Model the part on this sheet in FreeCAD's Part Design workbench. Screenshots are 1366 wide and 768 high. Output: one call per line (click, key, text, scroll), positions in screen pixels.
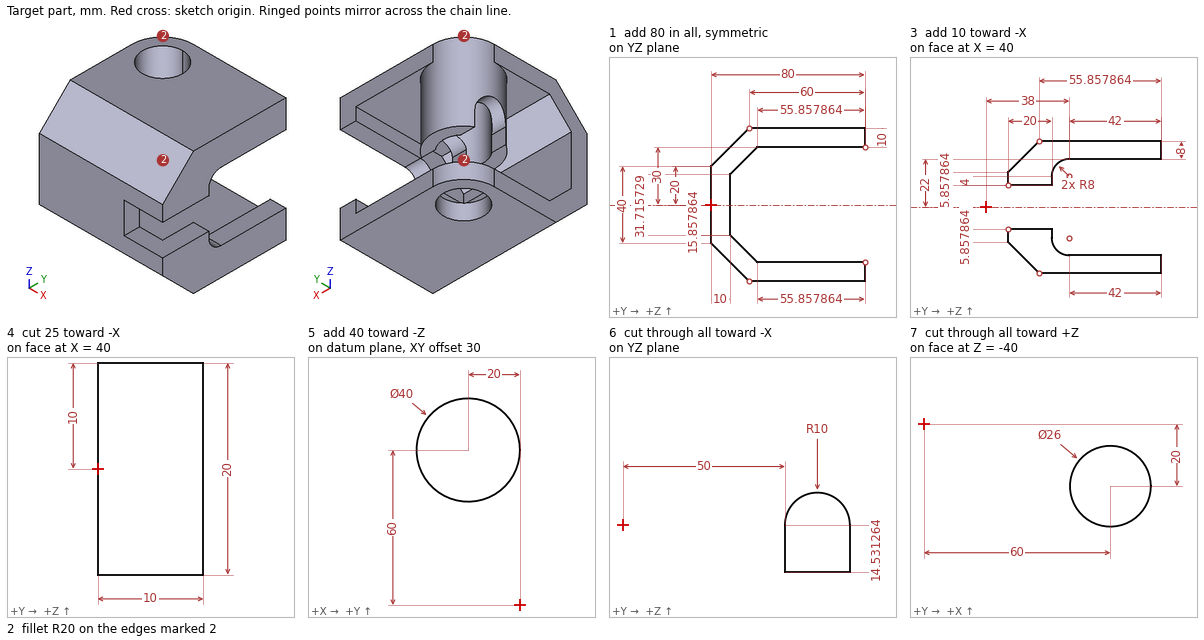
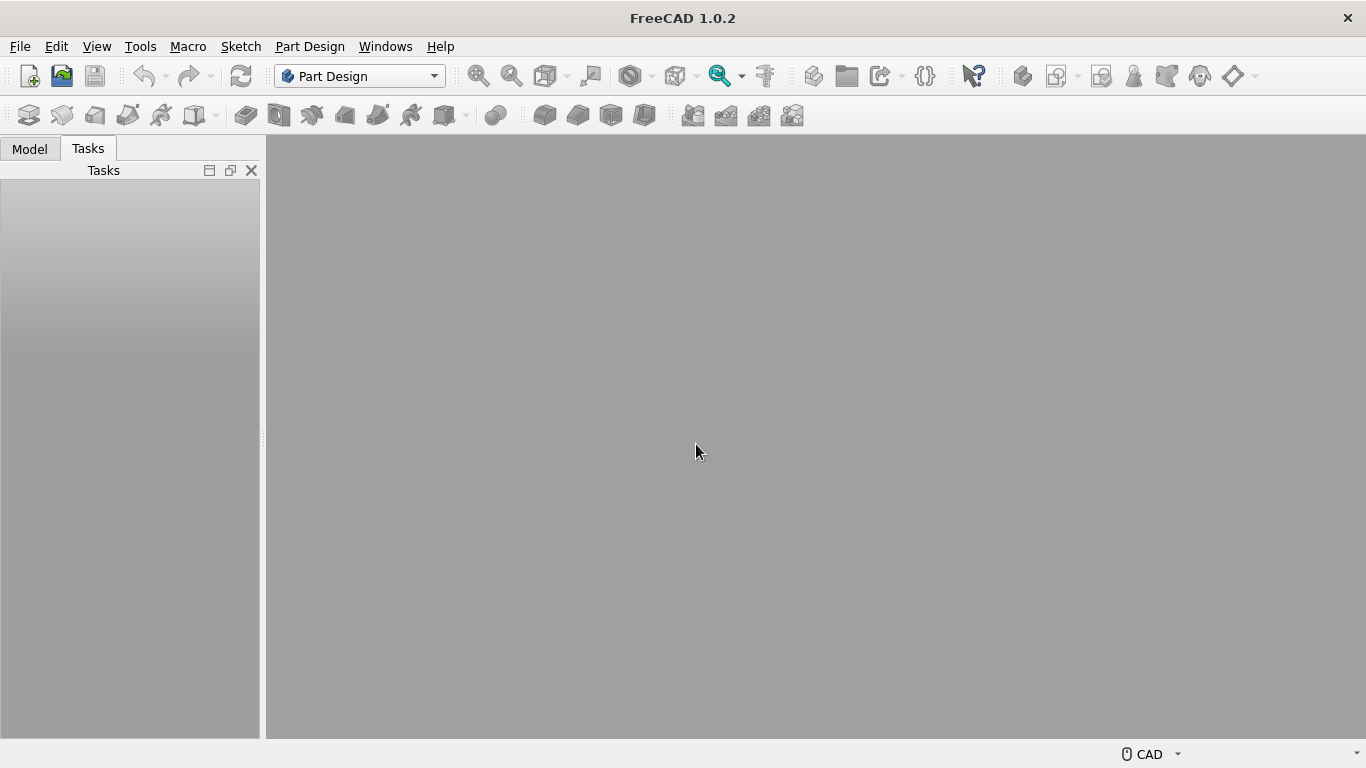
key(ctrl+n)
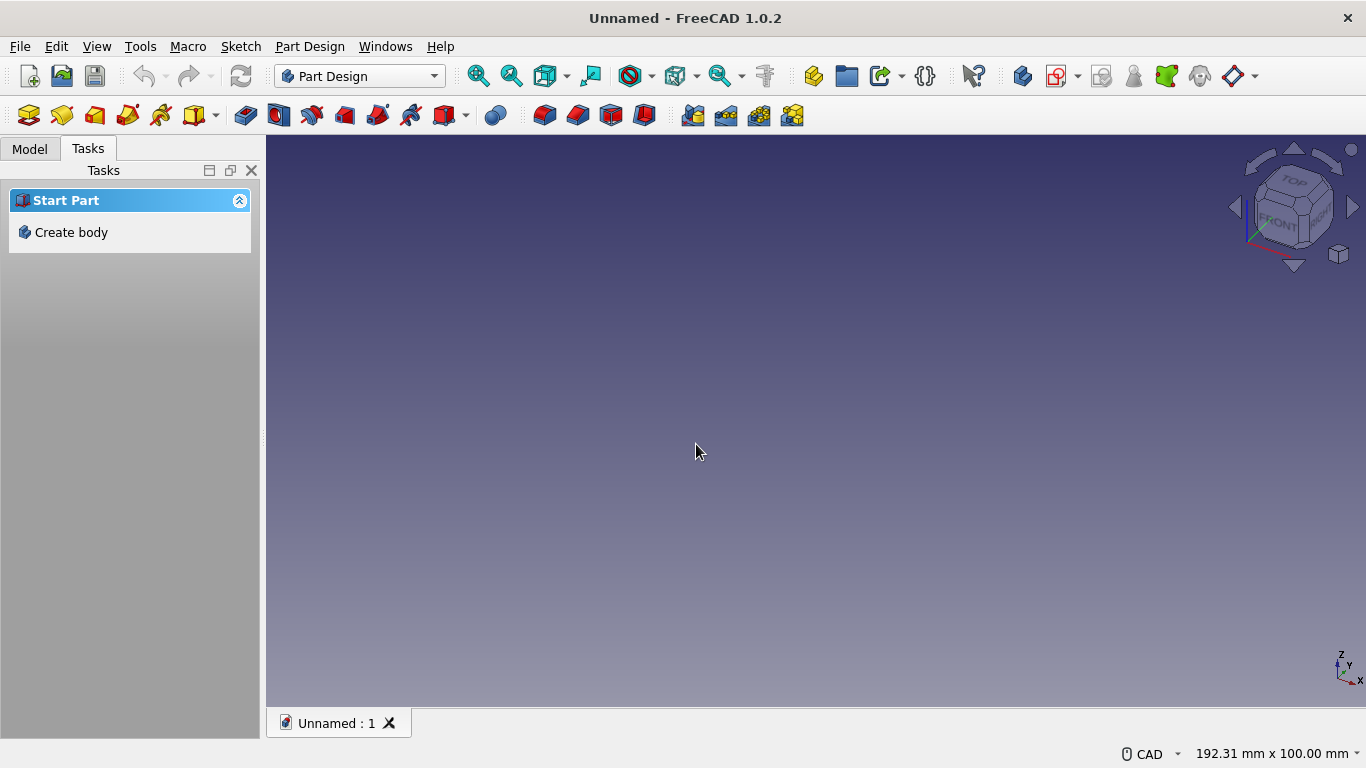
click(1056, 76)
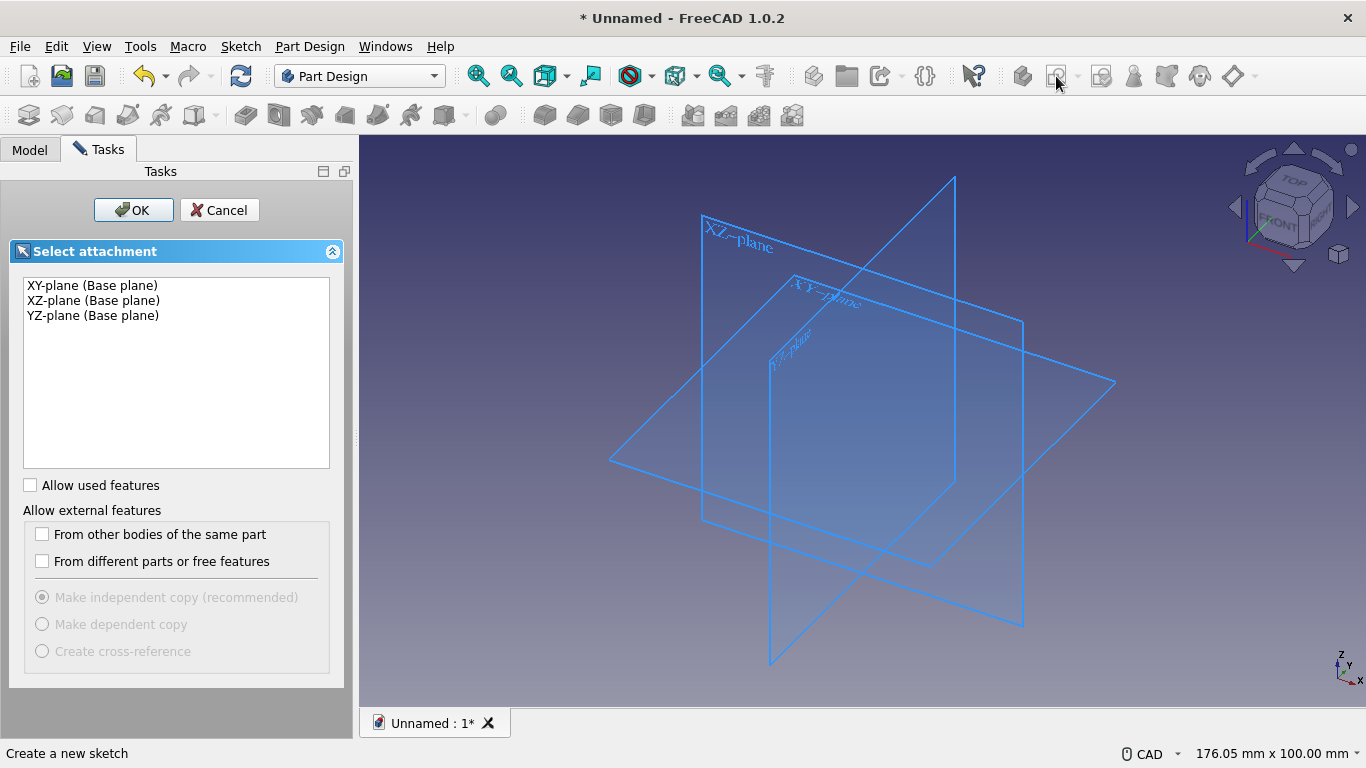
click(84, 316)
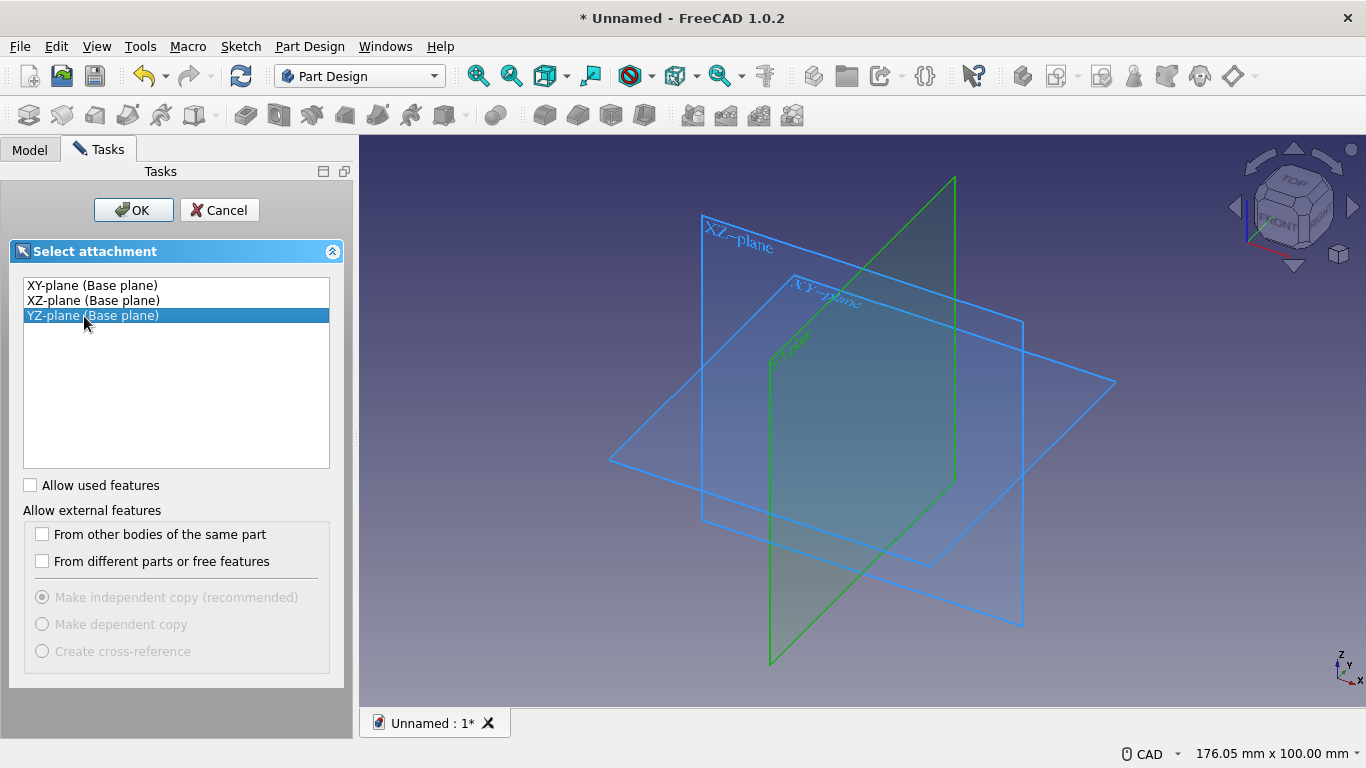
click(134, 210)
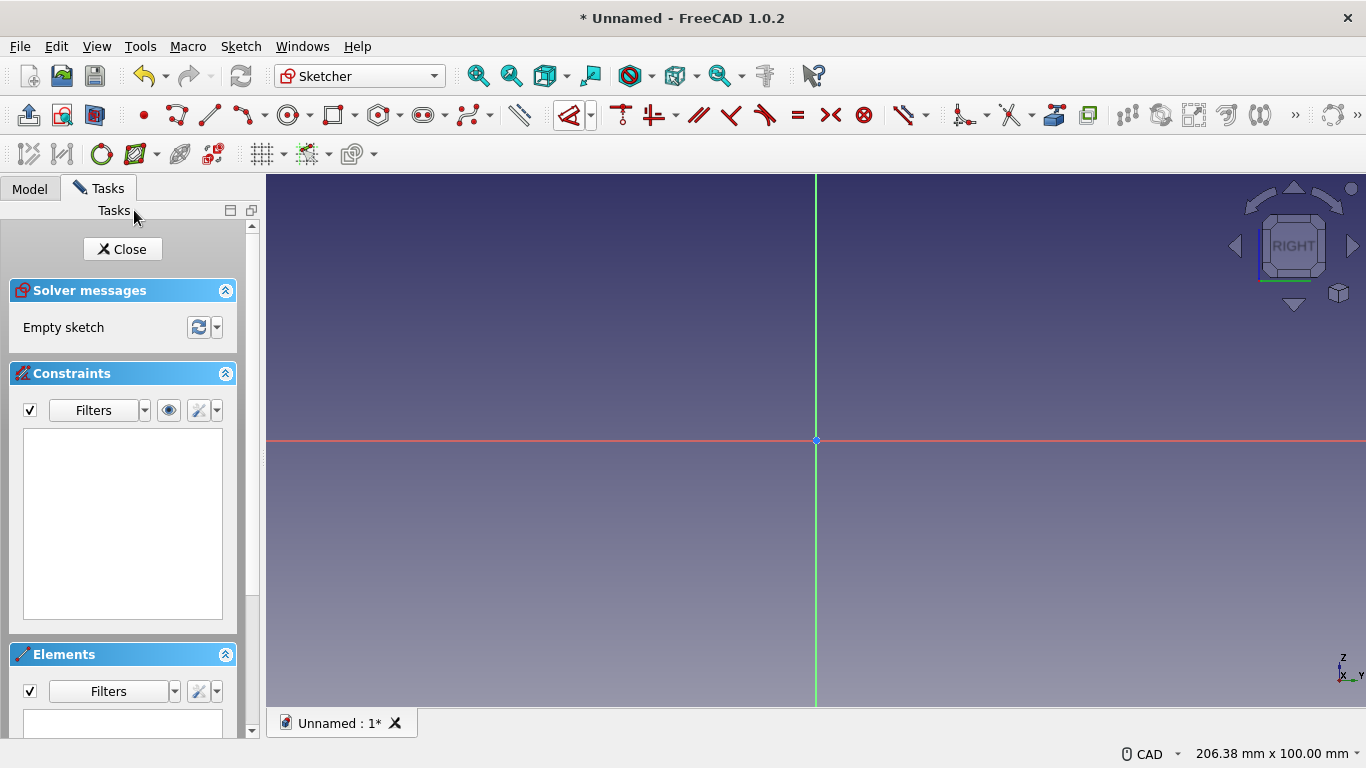
scroll(294, 440, down, 1)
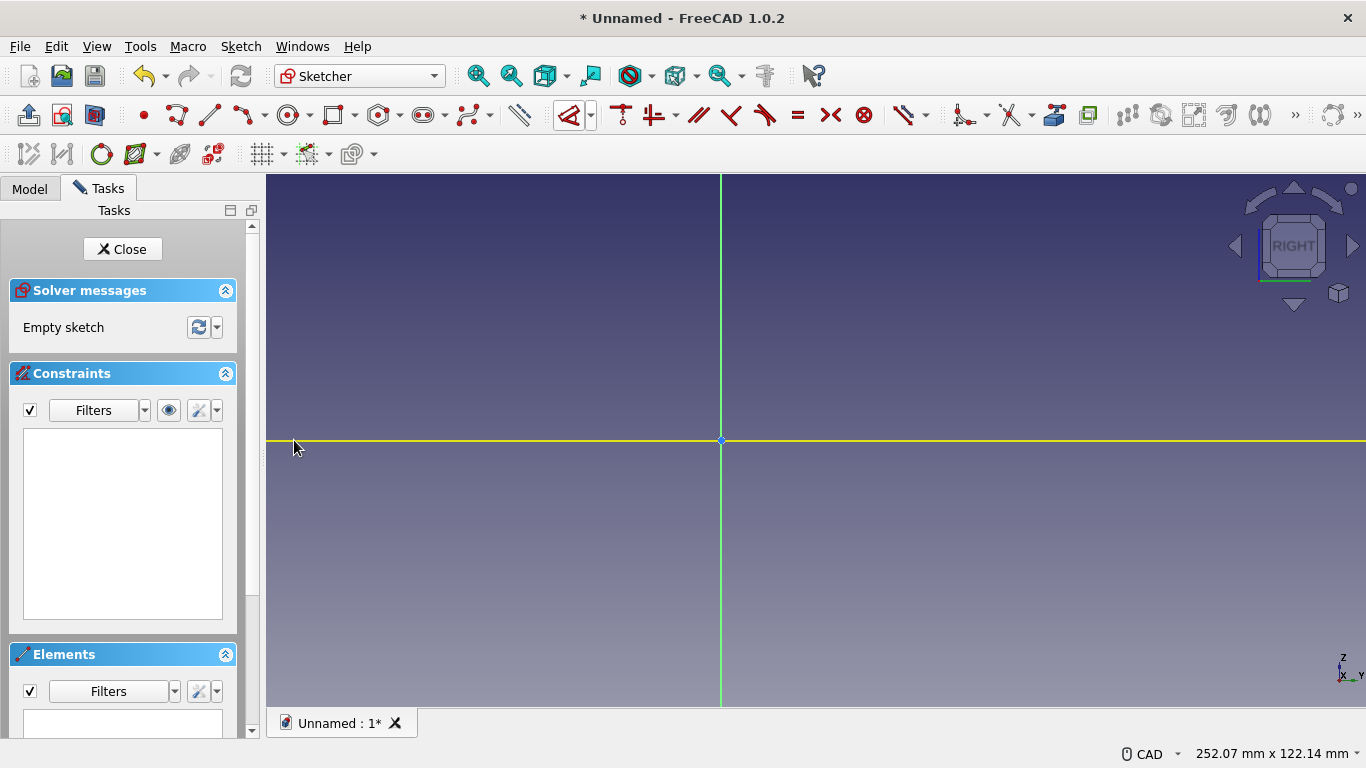
click(177, 116)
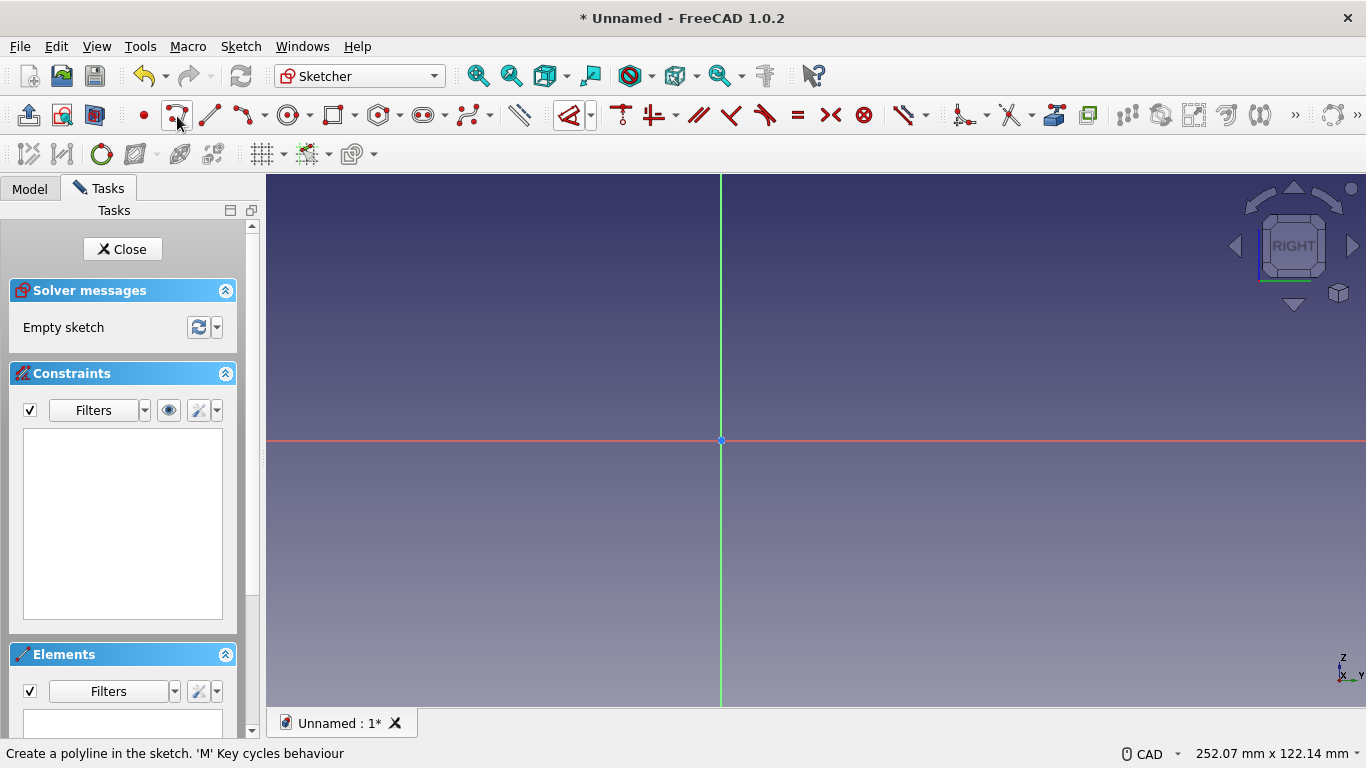
click(765, 510)
click(765, 371)
click(827, 310)
click(1070, 310)
click(1070, 266)
click(809, 266)
click(721, 353)
click(730, 528)
click(809, 615)
click(1070, 615)
click(1070, 571)
click(827, 571)
click(765, 511)
key(Escape)
key(Escape)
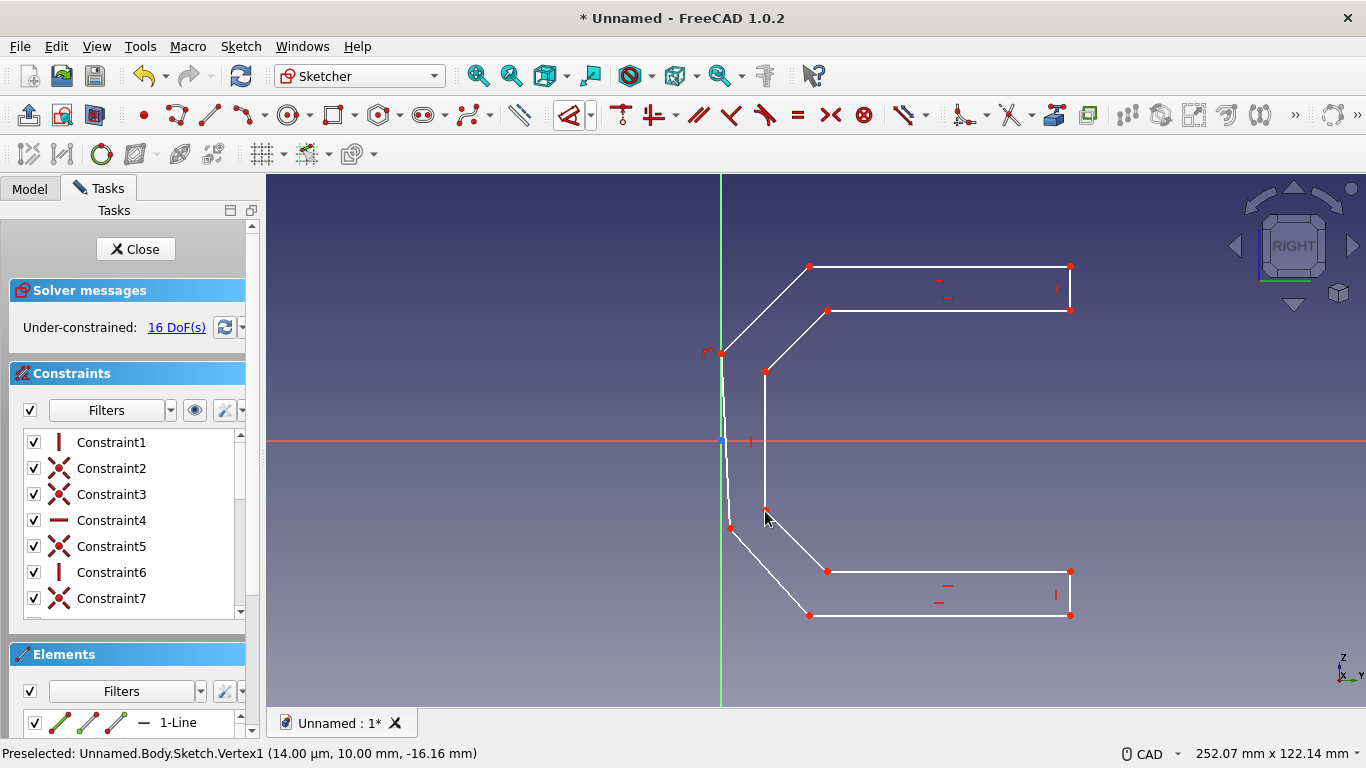
click(724, 407)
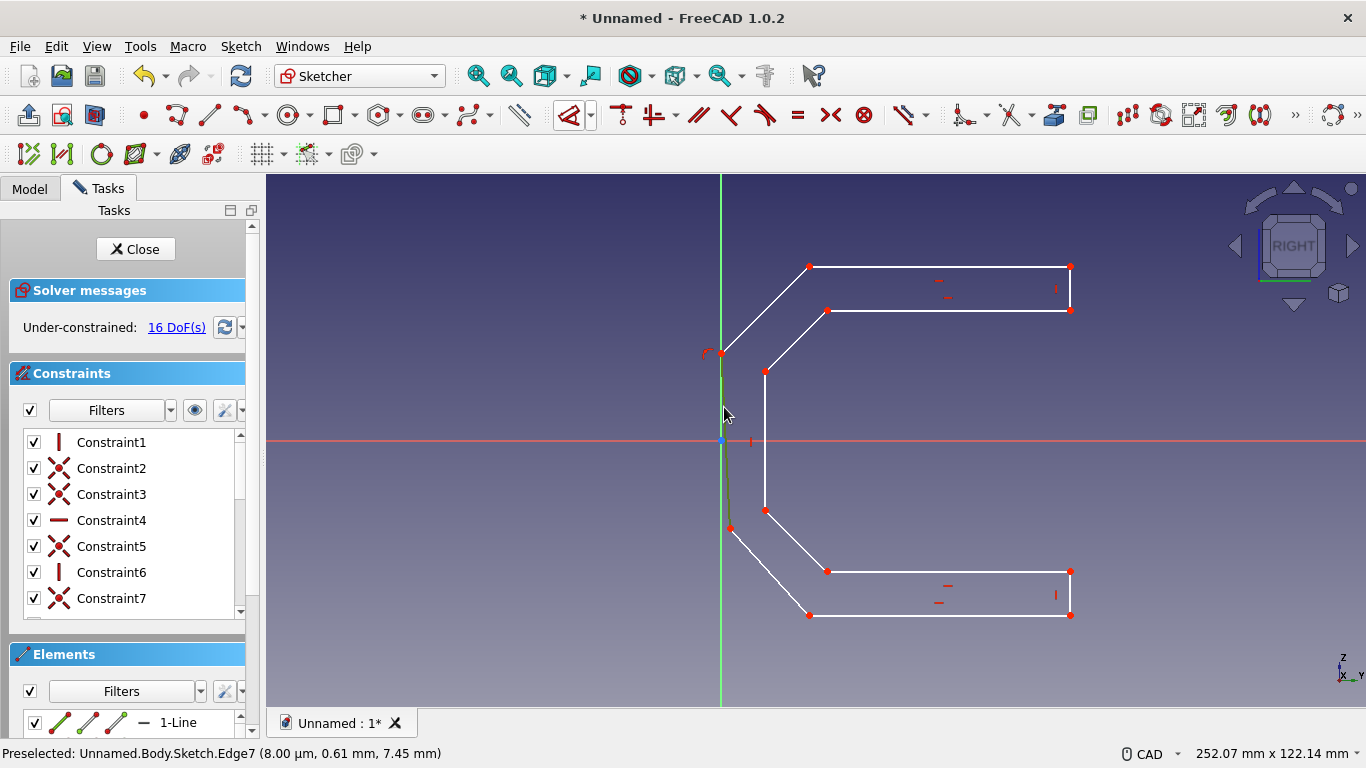
click(676, 116)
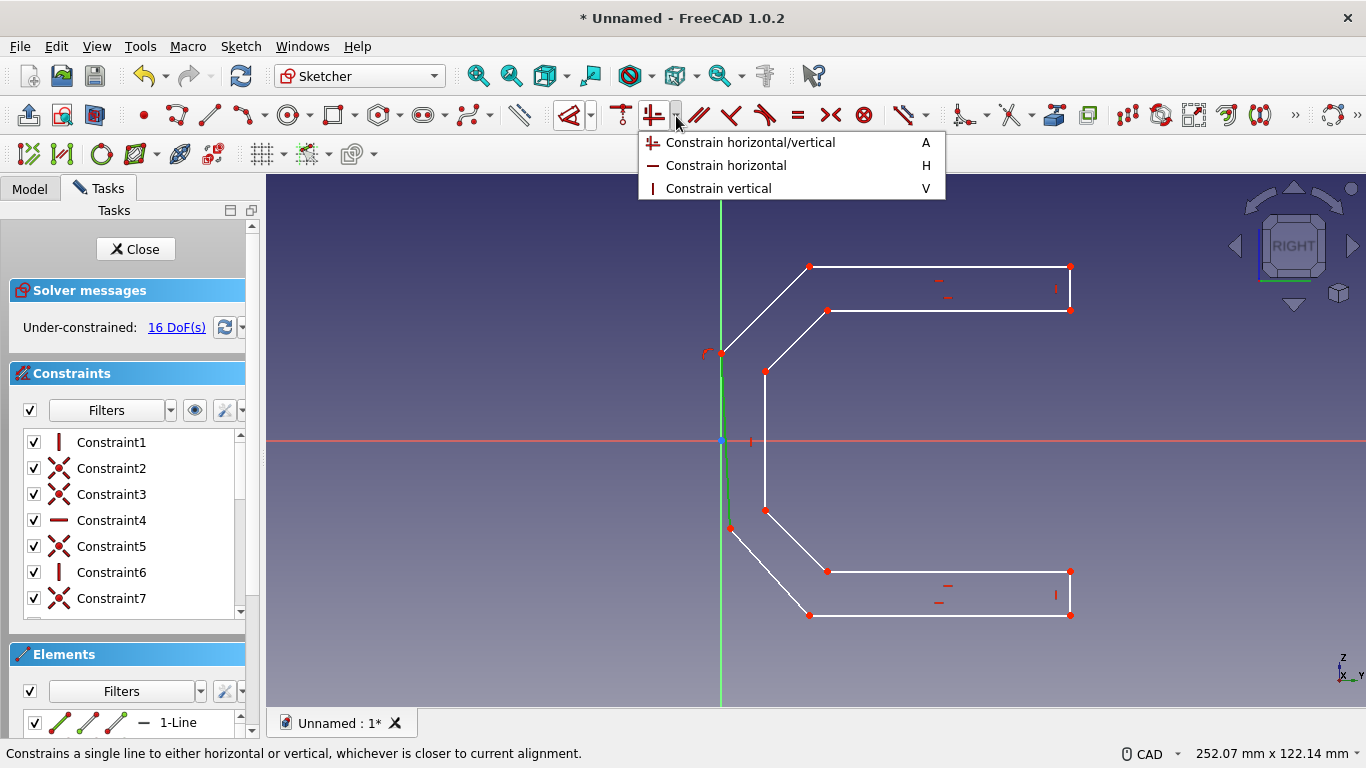
click(792, 188)